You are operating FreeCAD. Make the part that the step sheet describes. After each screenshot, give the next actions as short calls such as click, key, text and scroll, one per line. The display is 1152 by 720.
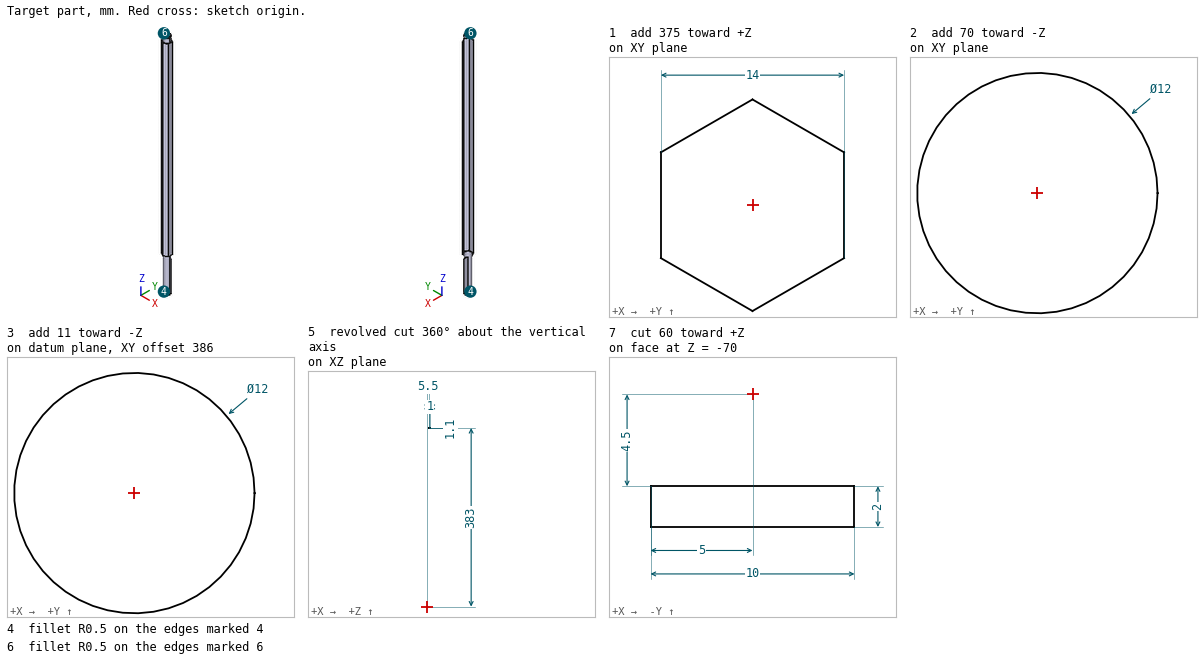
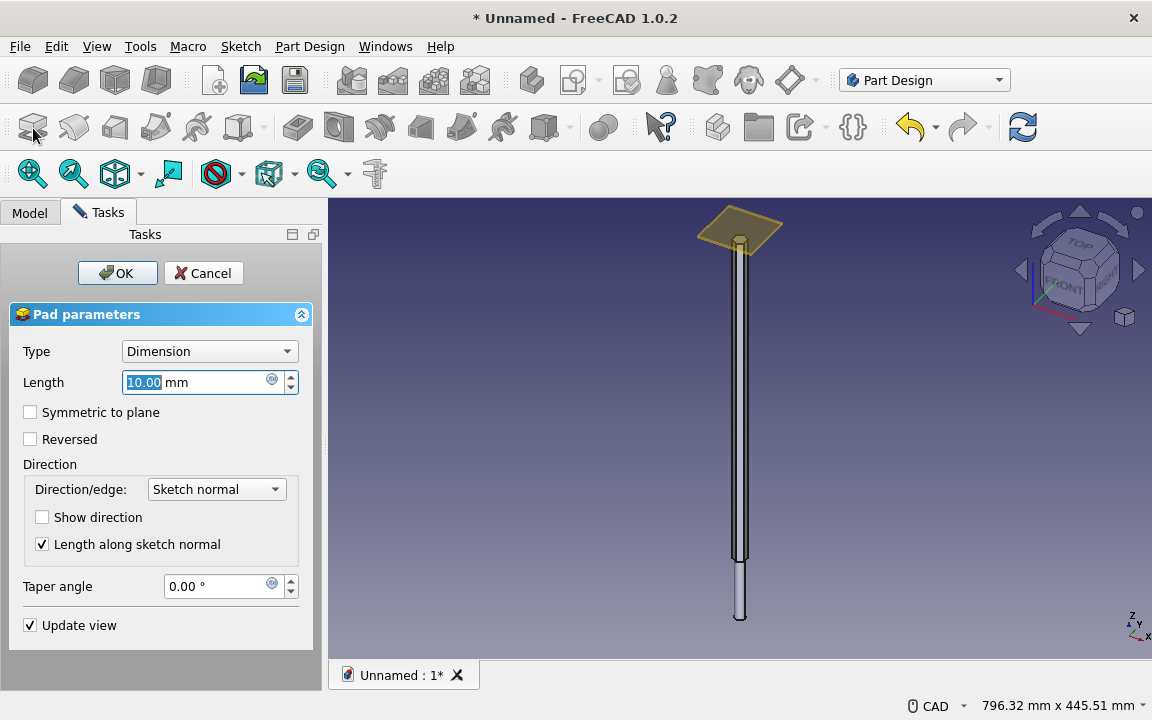
text(11)
key(Tab)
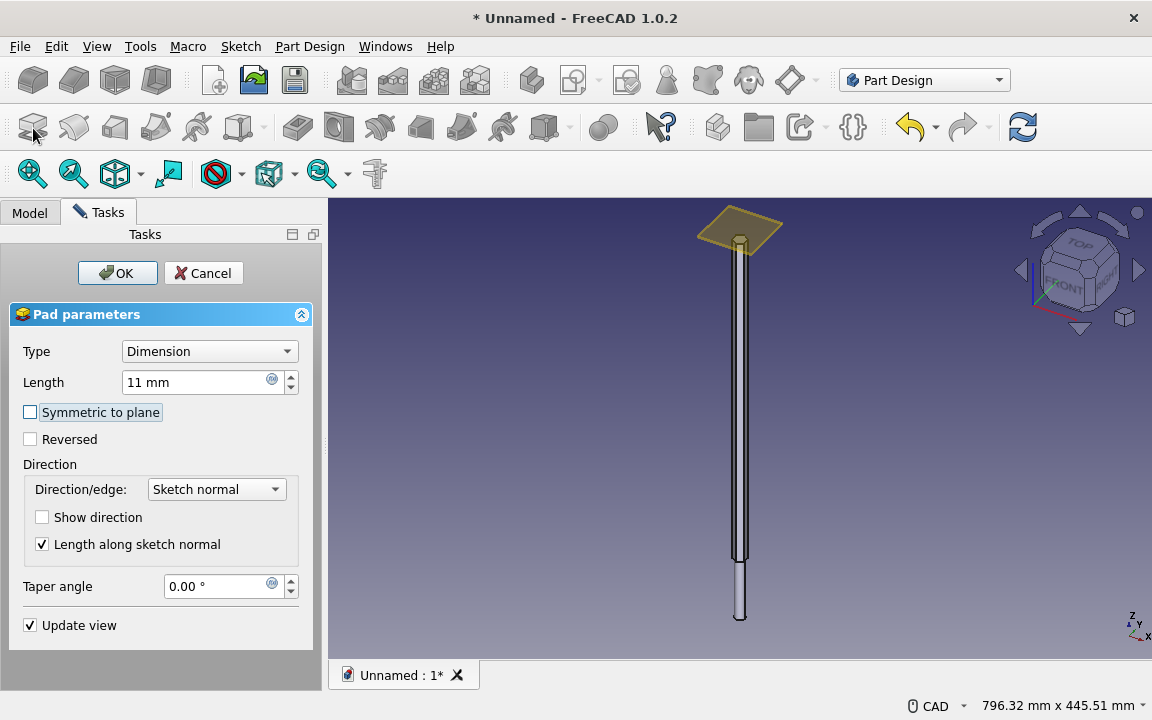
click(31, 439)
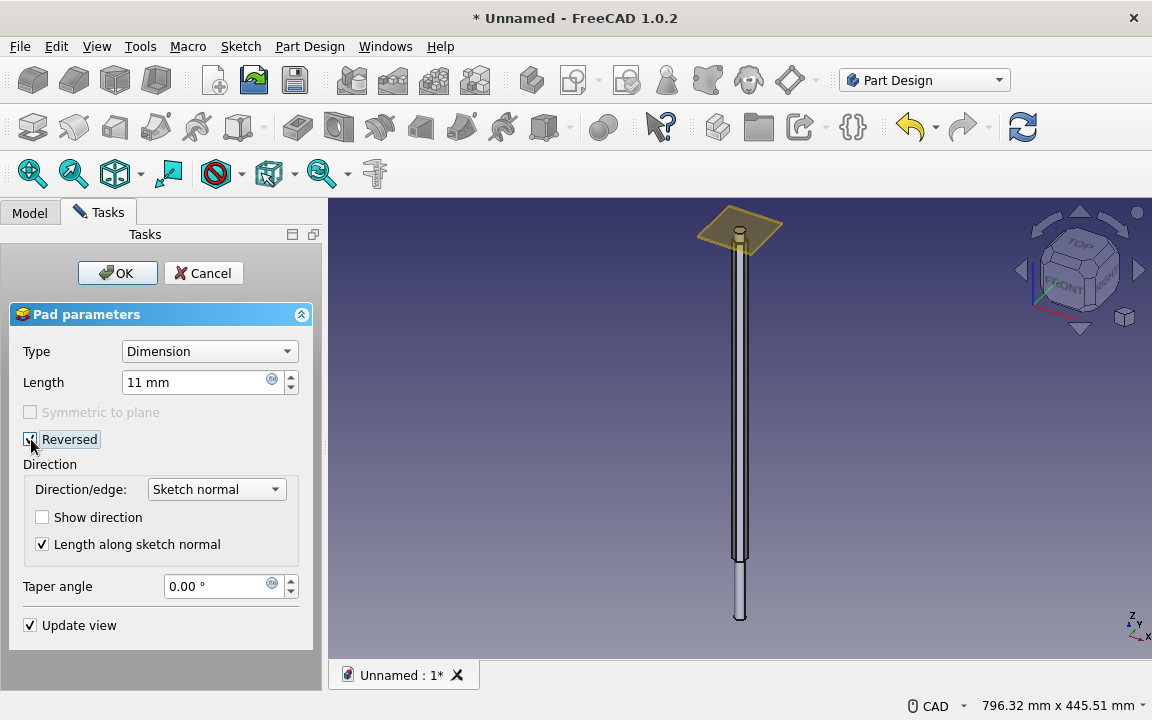
click(118, 273)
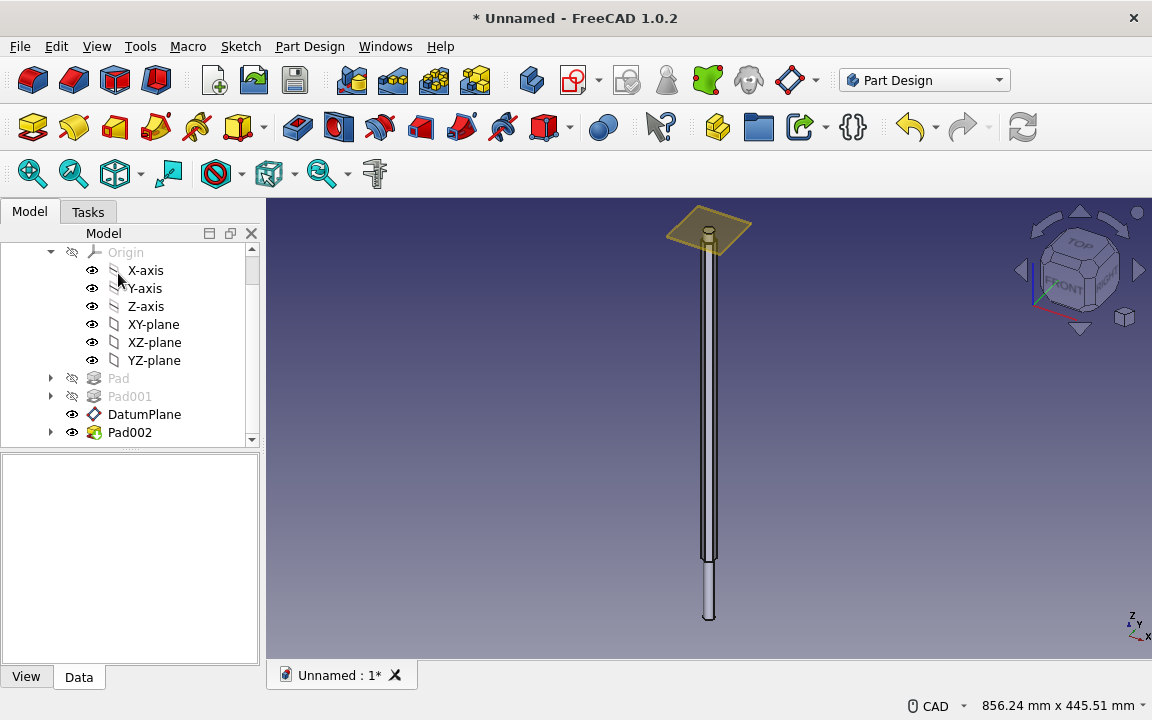
click(117, 414)
key(space)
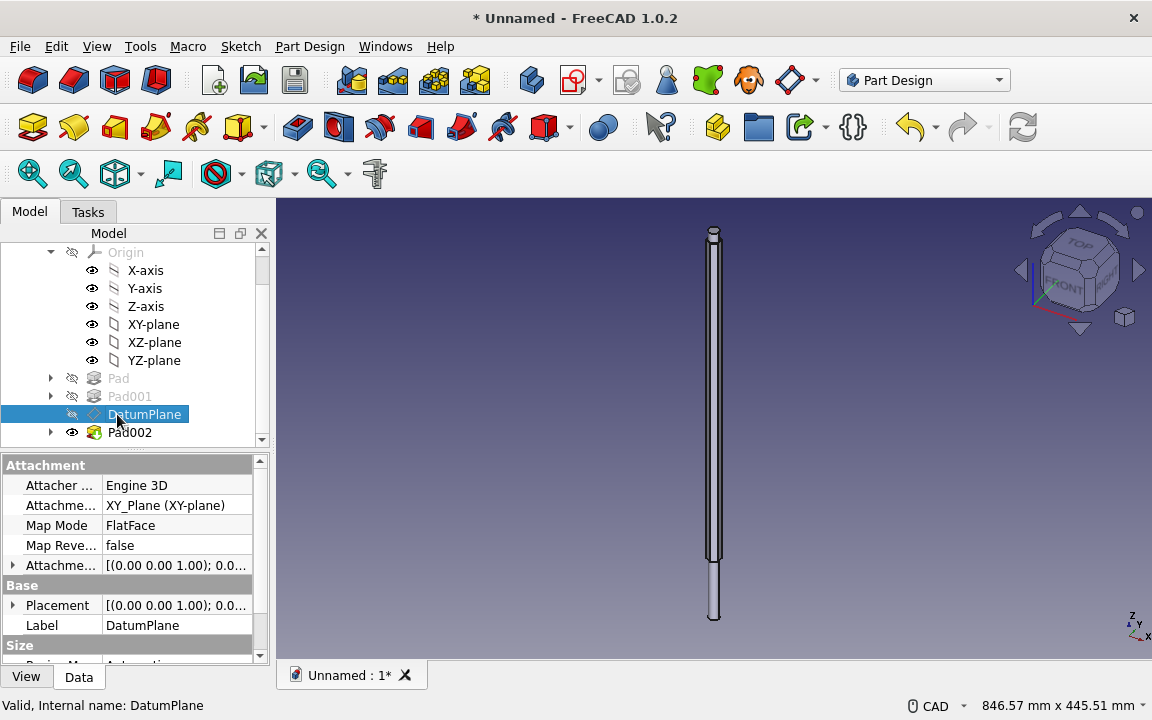
click(709, 618)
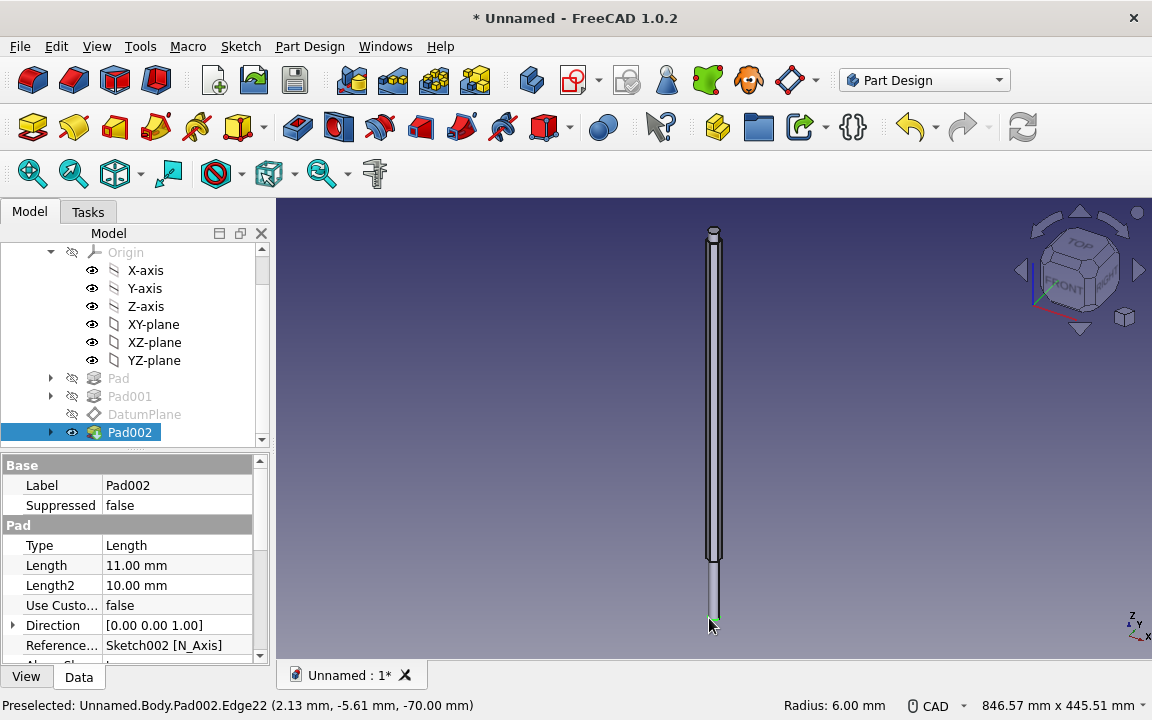
click(33, 80)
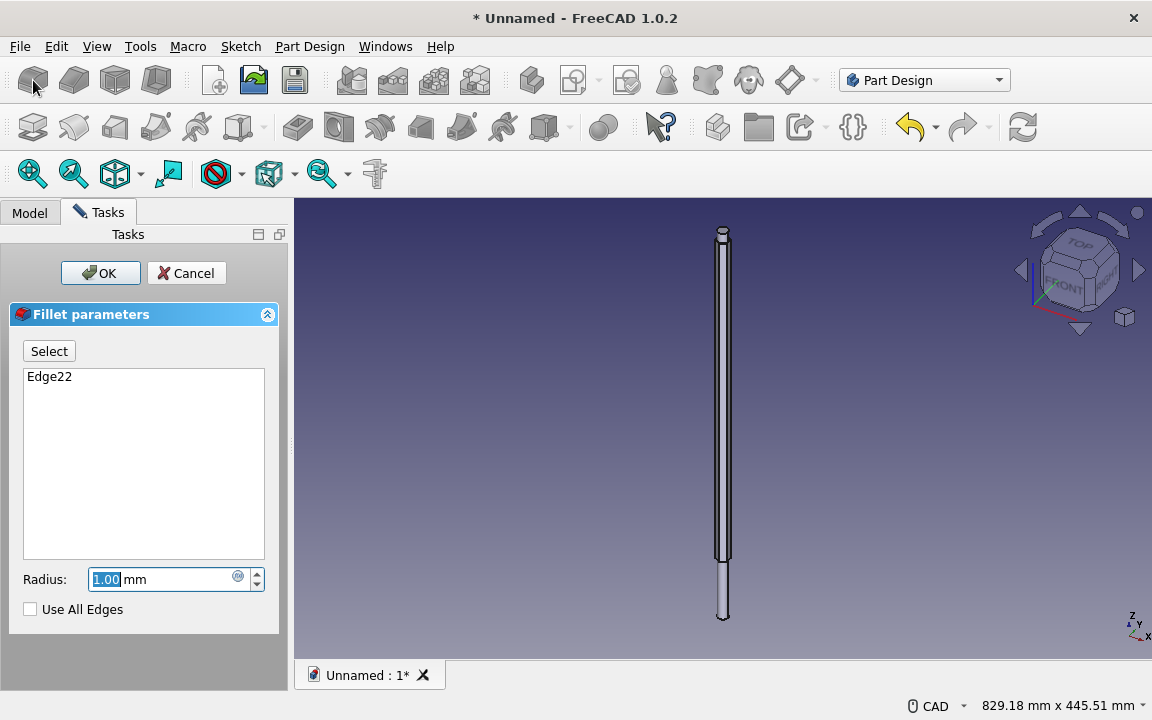
text(0.5)
key(Tab)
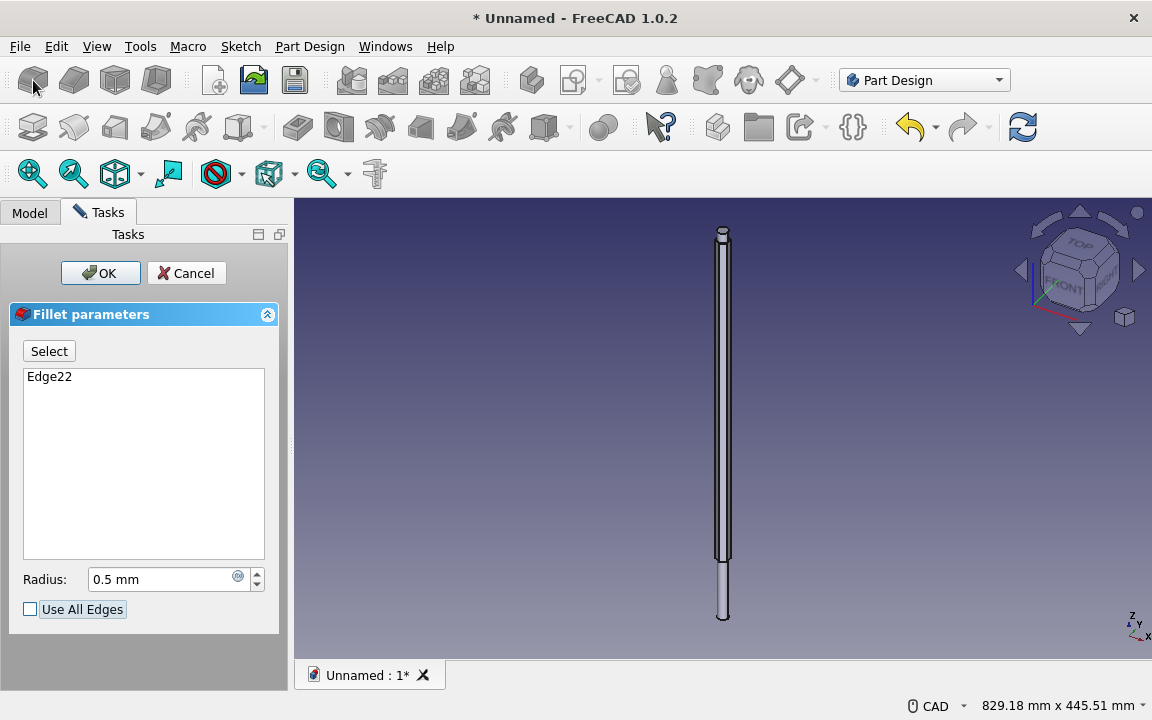
click(101, 273)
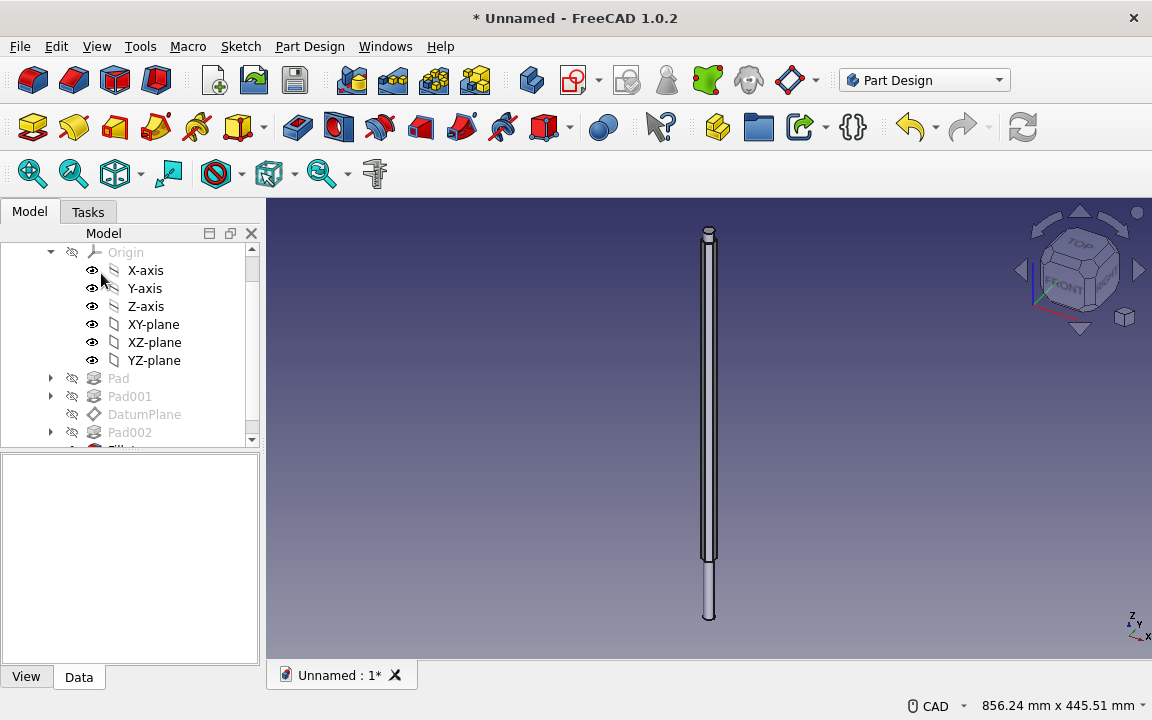
click(572, 80)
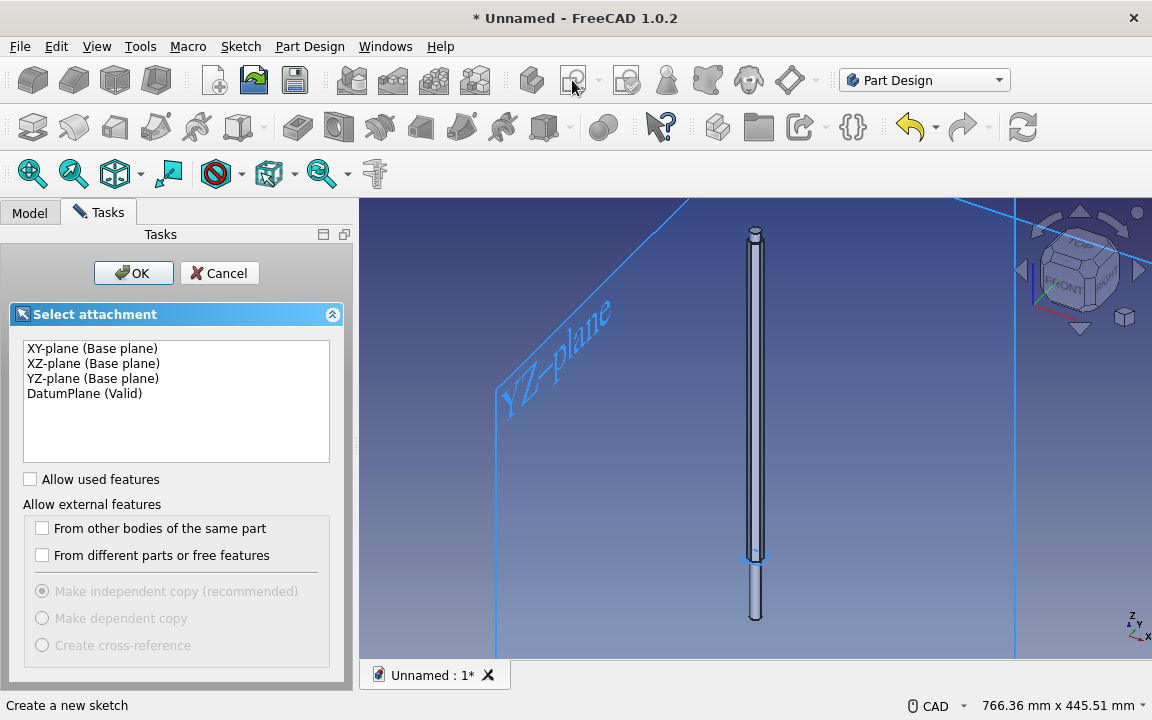
click(84, 364)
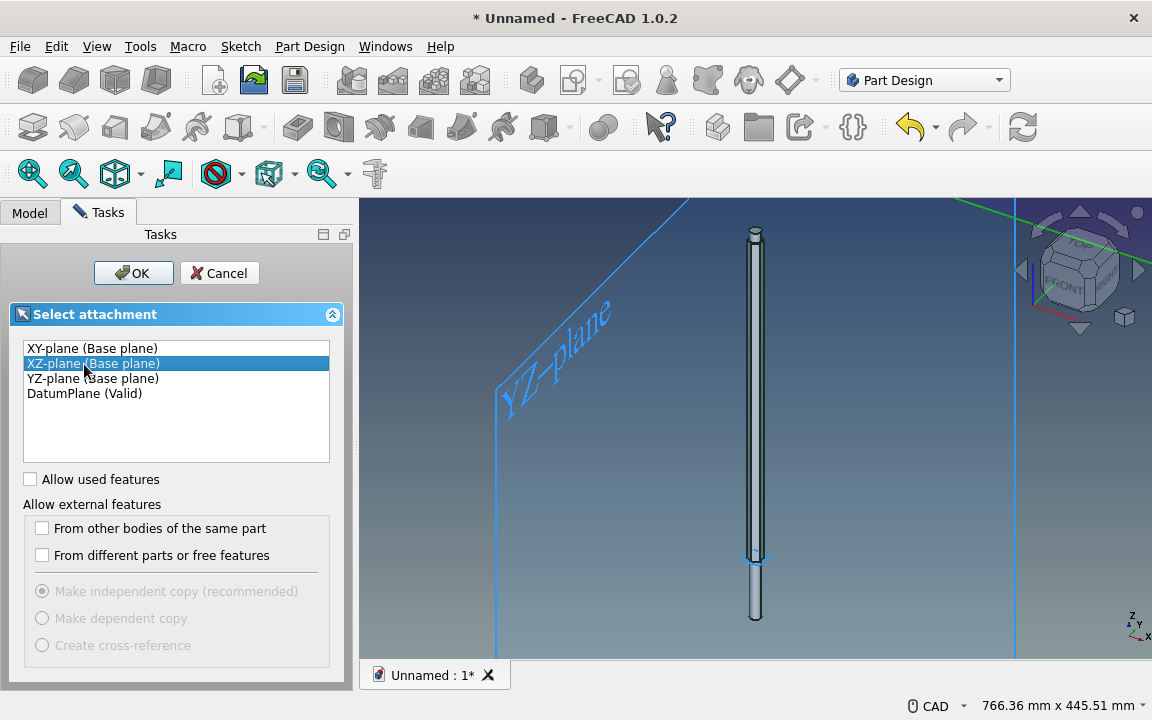
click(134, 273)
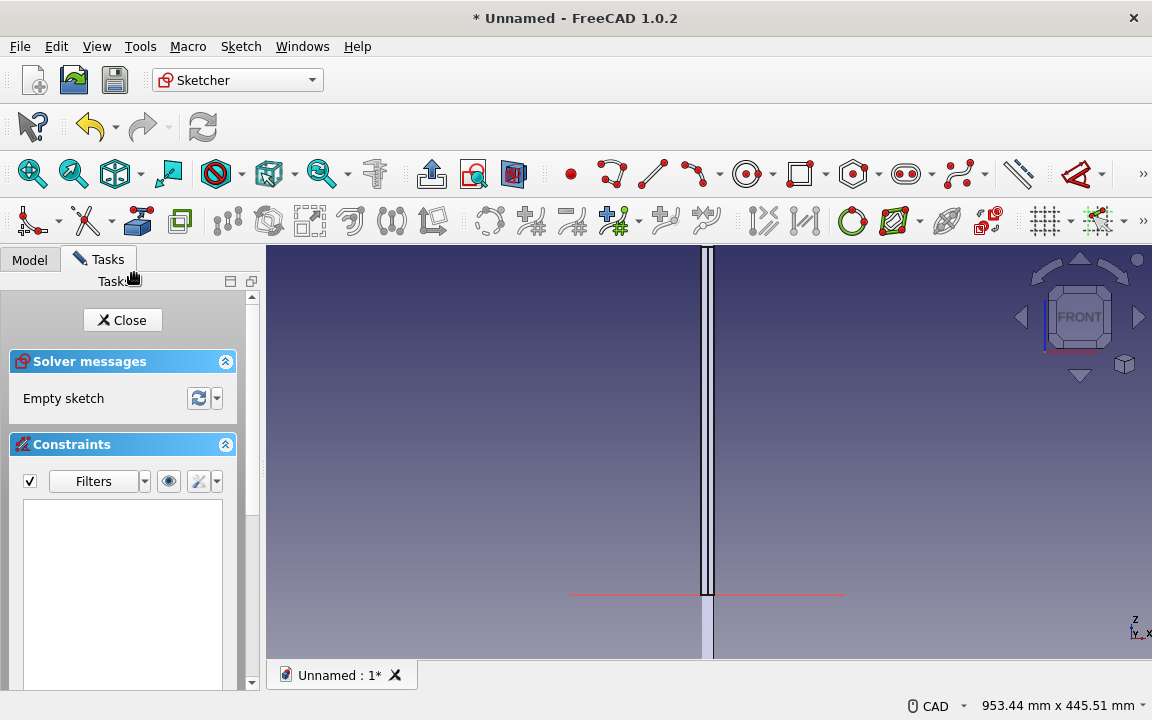
click(514, 174)